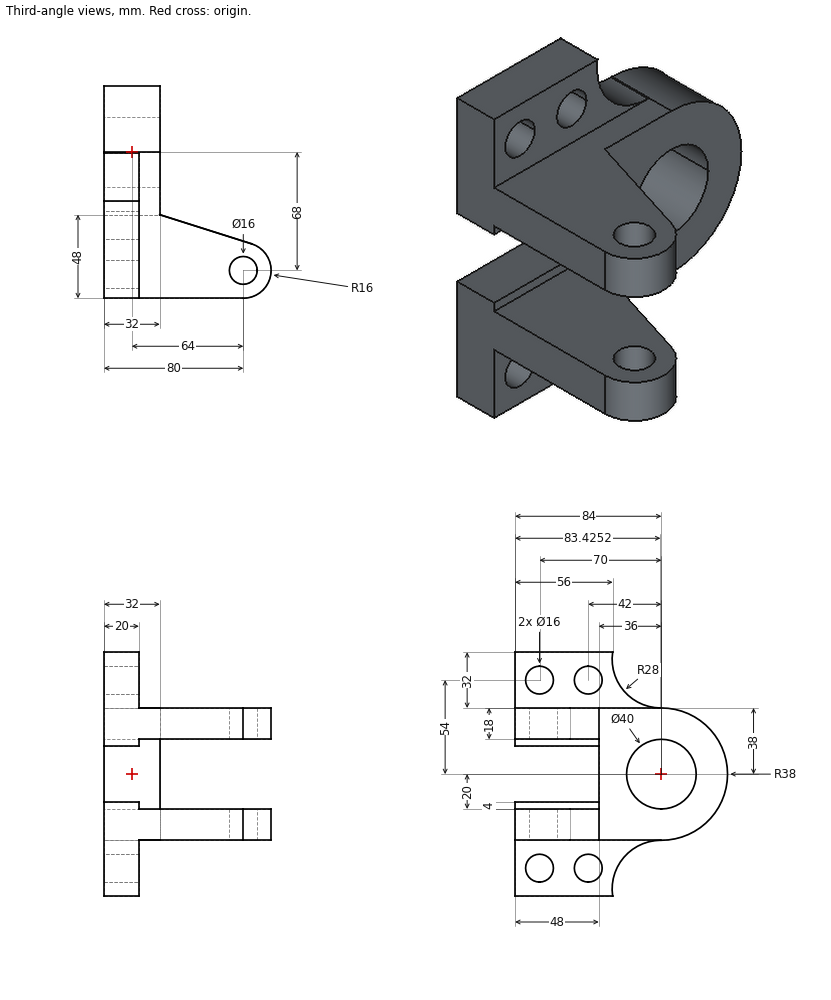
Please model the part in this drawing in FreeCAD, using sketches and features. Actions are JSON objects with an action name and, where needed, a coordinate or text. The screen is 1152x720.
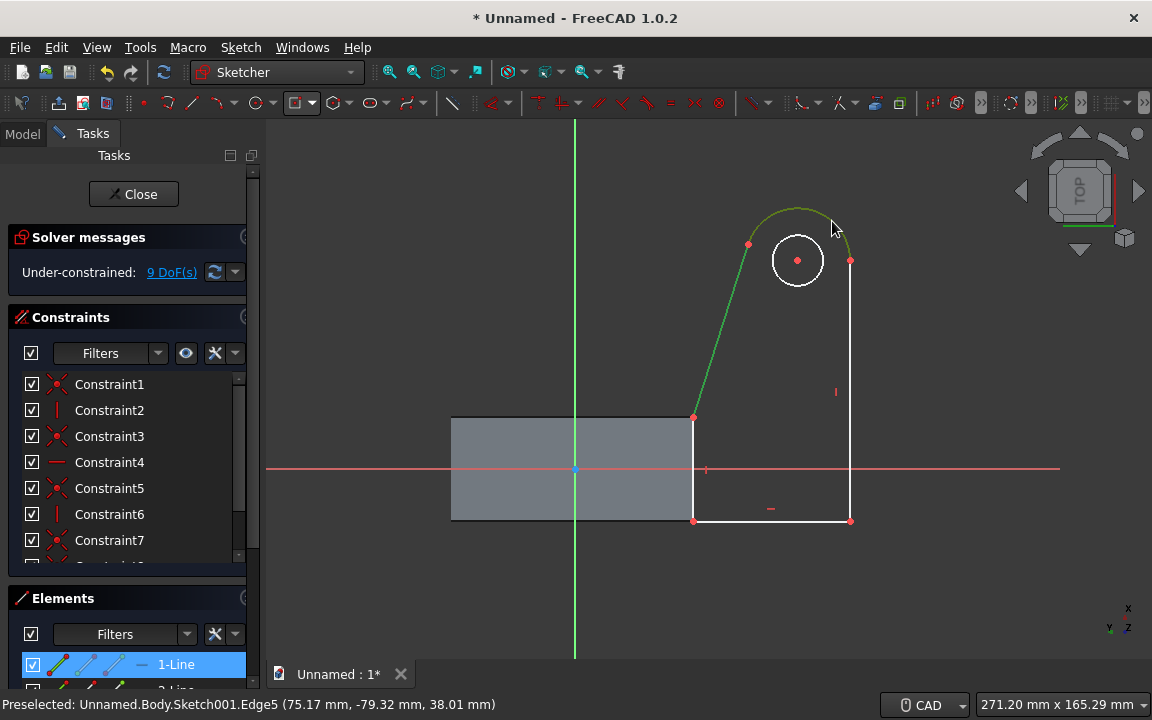
{"action": "left_click", "coordinate": [648, 104]}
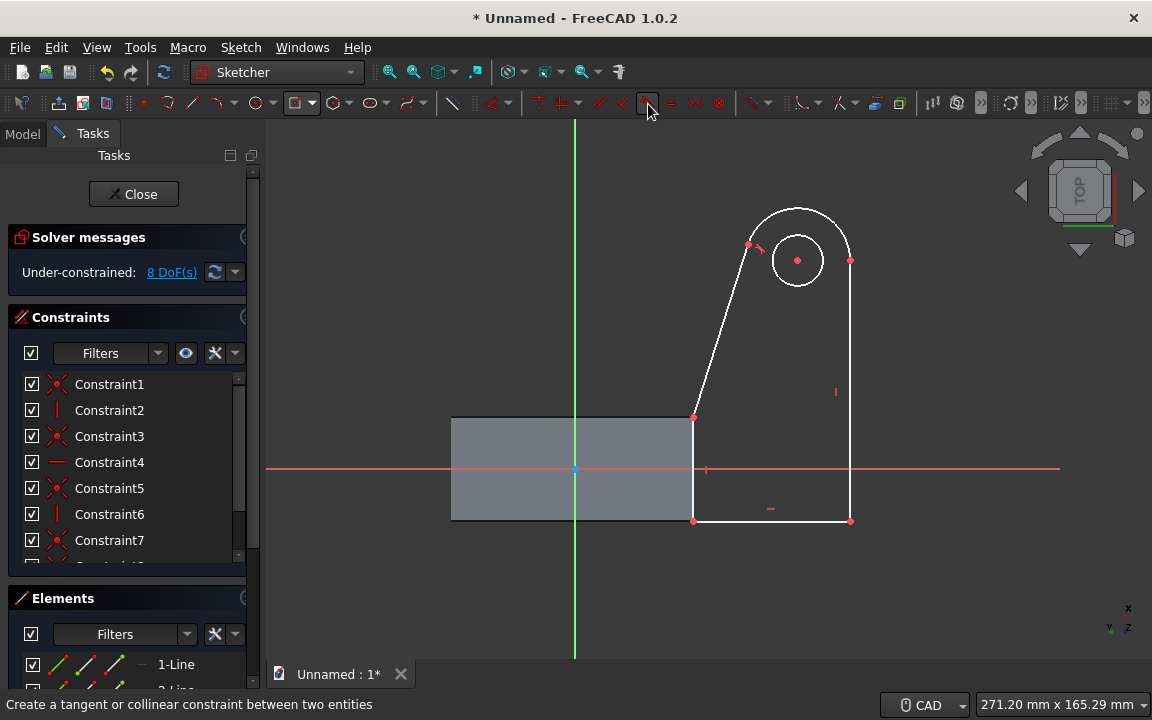
{"action": "left_click", "coordinate": [850, 444]}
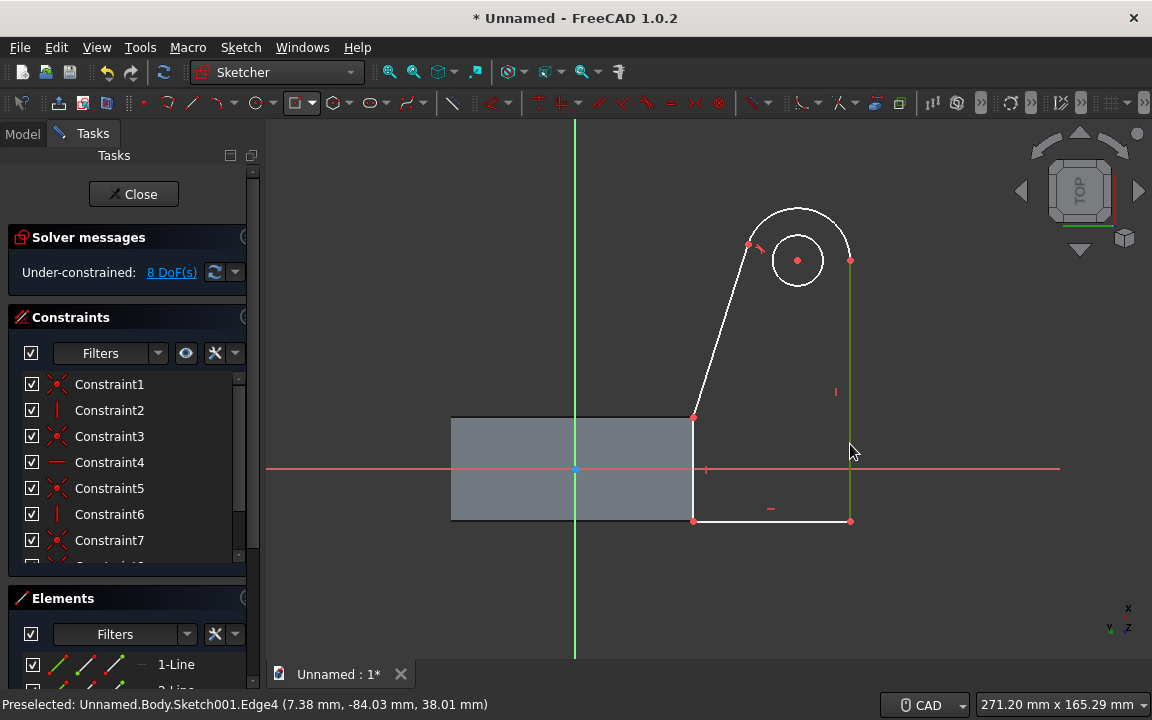
{"action": "left_click", "coordinate": [832, 222]}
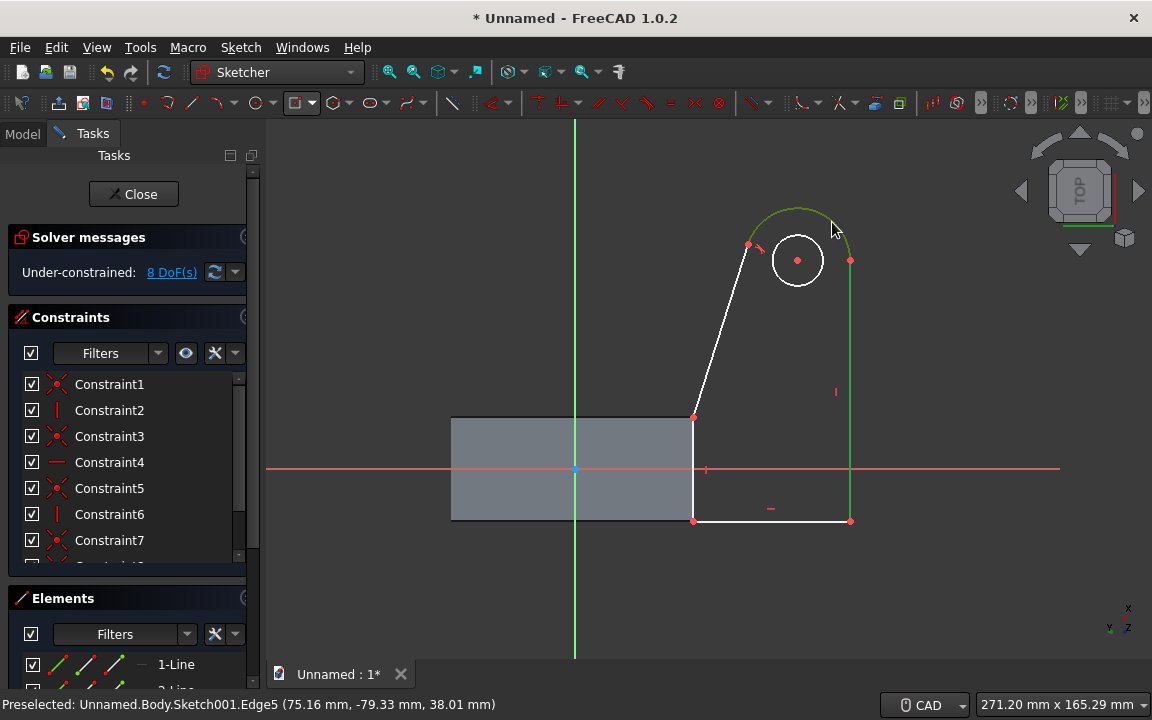
{"action": "left_click", "coordinate": [648, 104]}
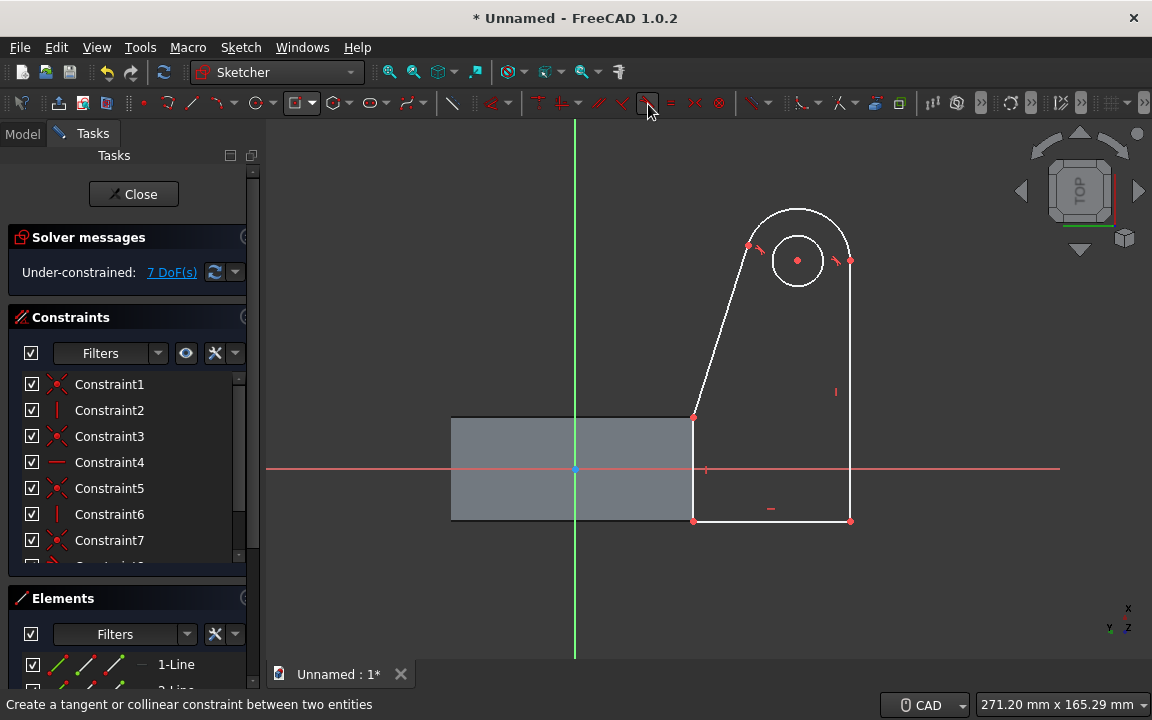
{"action": "left_click", "coordinate": [492, 104]}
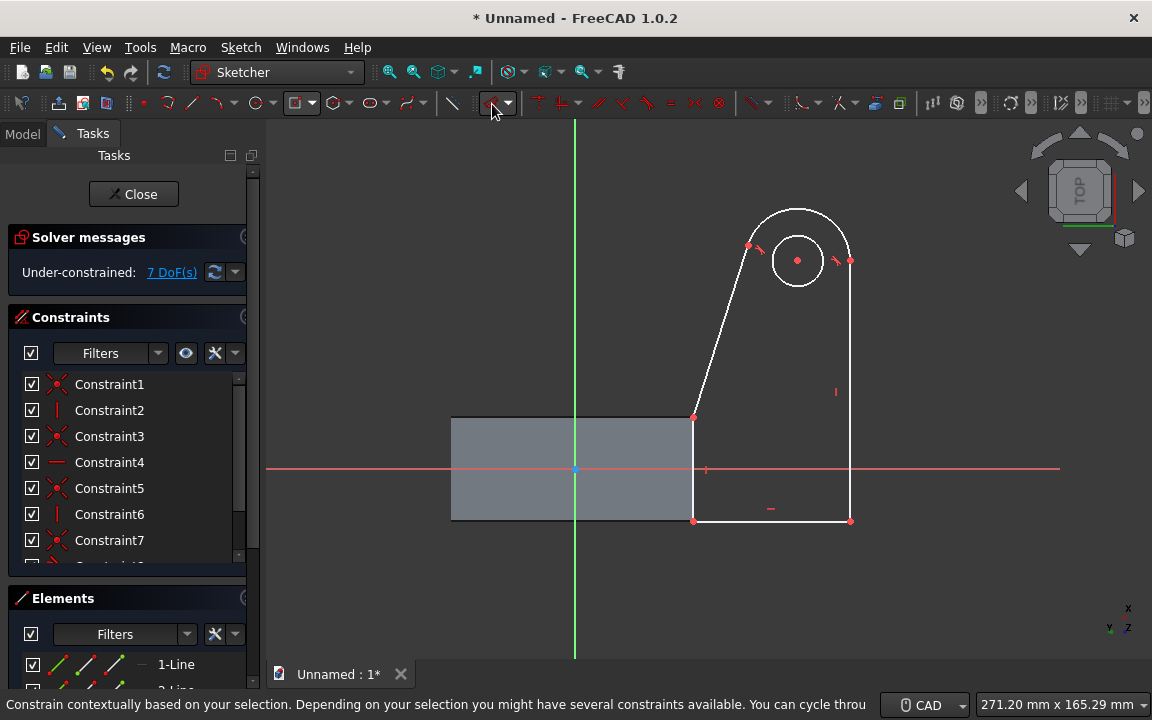
{"action": "left_click", "coordinate": [832, 222]}
{"action": "left_click", "coordinate": [853, 198]}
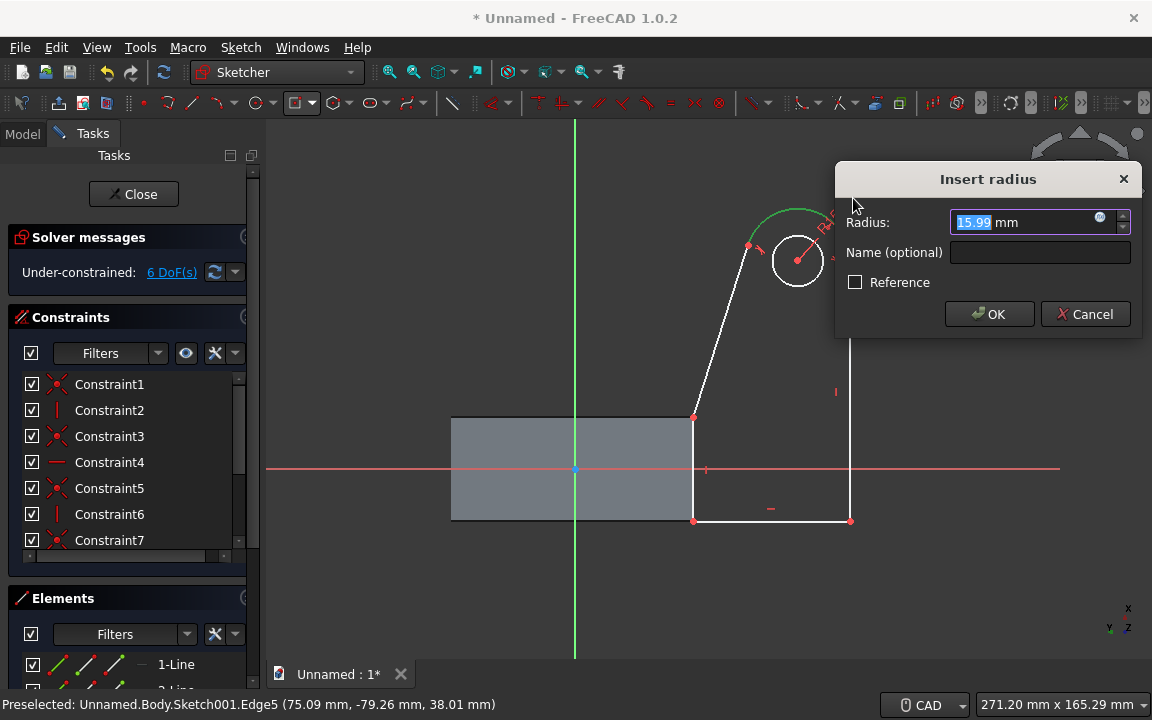
{"action": "type", "text": "16"}
{"action": "key", "text": "Return"}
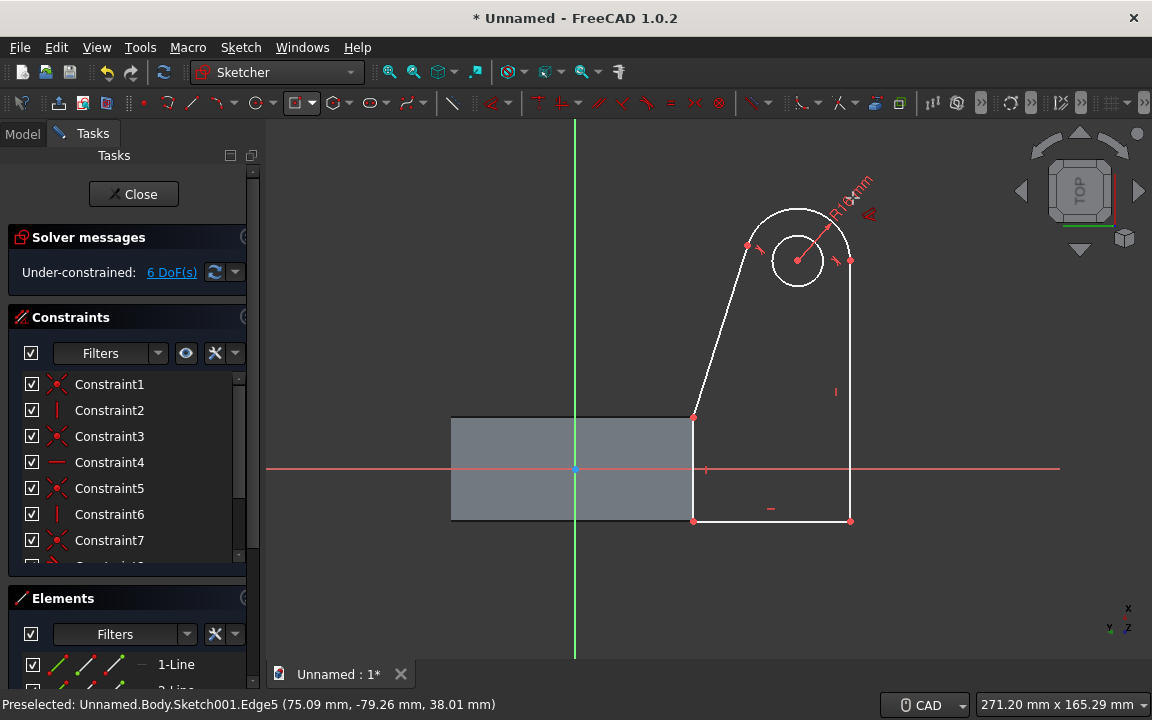
{"action": "left_click", "coordinate": [816, 243]}
{"action": "left_click", "coordinate": [757, 302]}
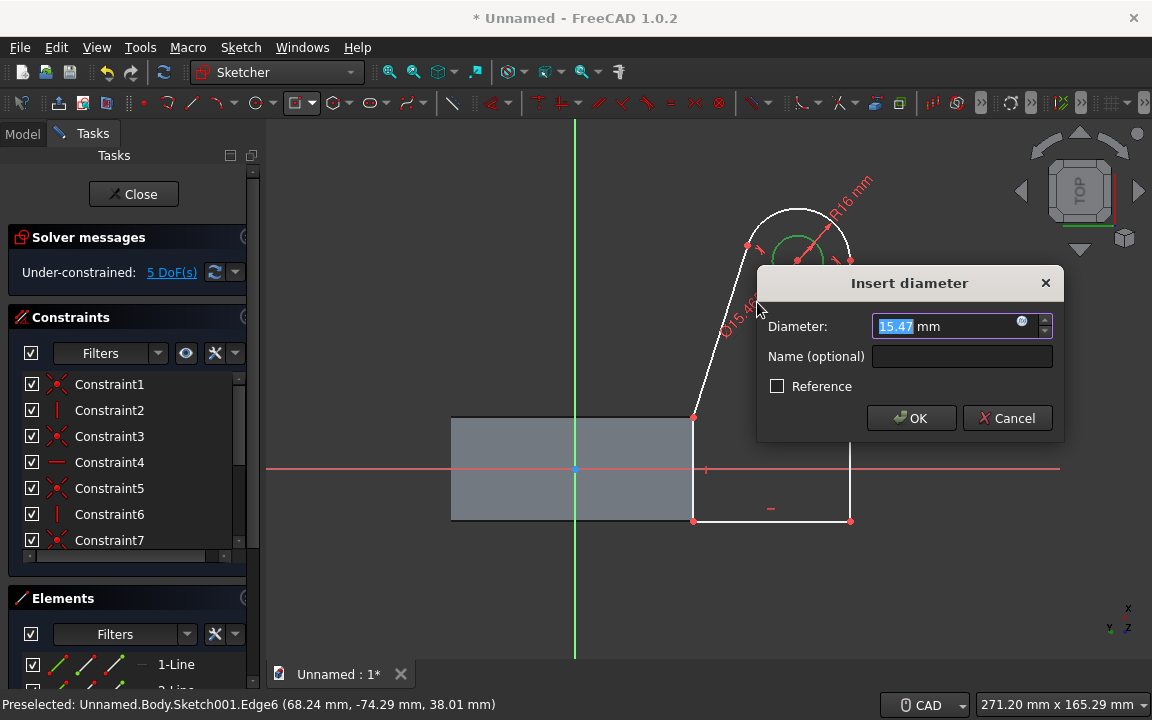
{"action": "type", "text": "16"}
{"action": "key", "text": "Return"}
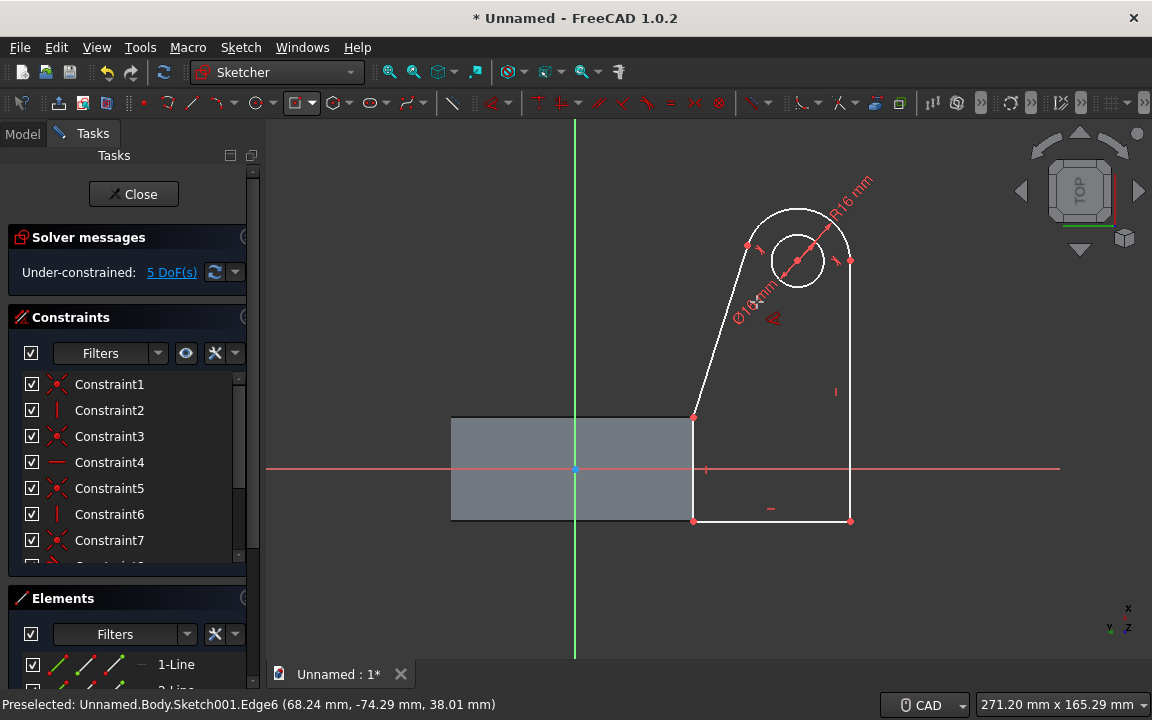
{"action": "left_click", "coordinate": [693, 449]}
{"action": "left_click", "coordinate": [659, 446]}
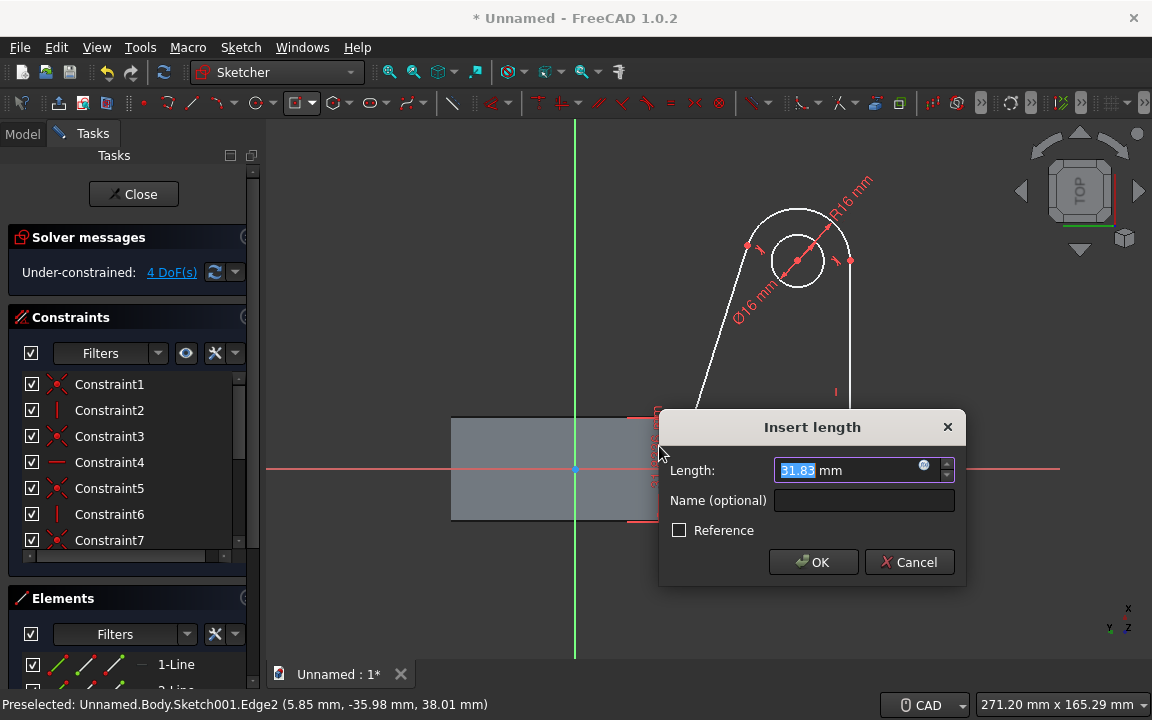
{"action": "type", "text": "32"}
{"action": "key", "text": "Return"}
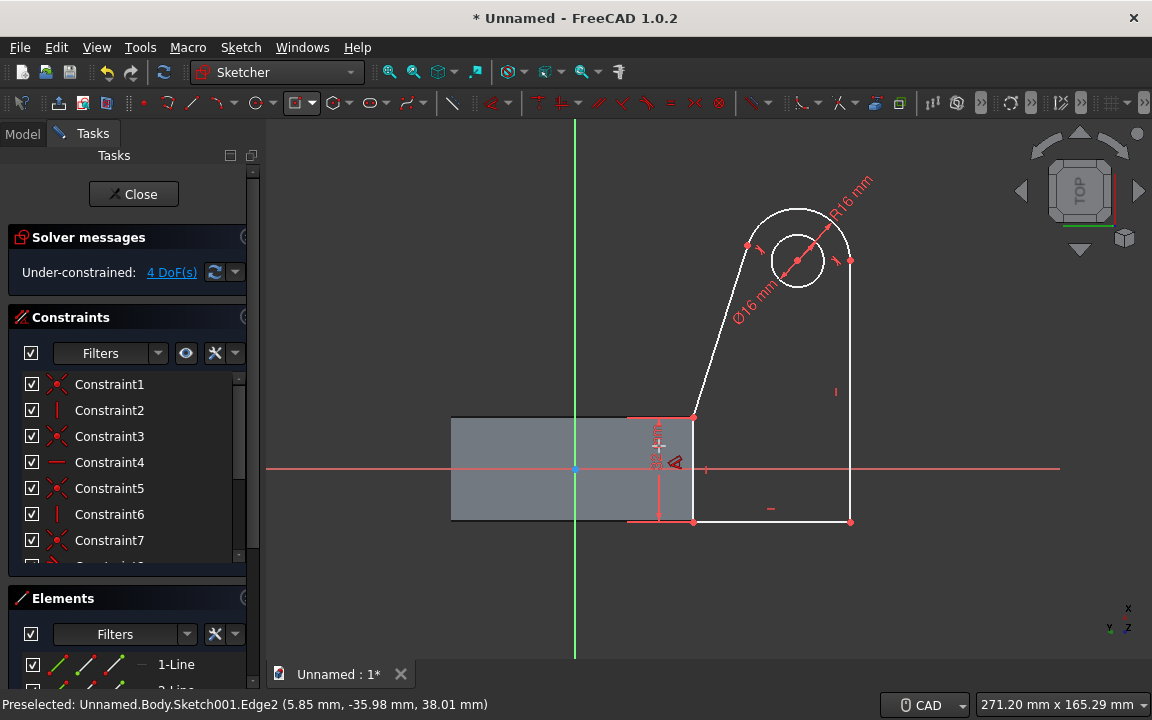
{"action": "left_click", "coordinate": [740, 522]}
{"action": "left_click", "coordinate": [772, 556]}